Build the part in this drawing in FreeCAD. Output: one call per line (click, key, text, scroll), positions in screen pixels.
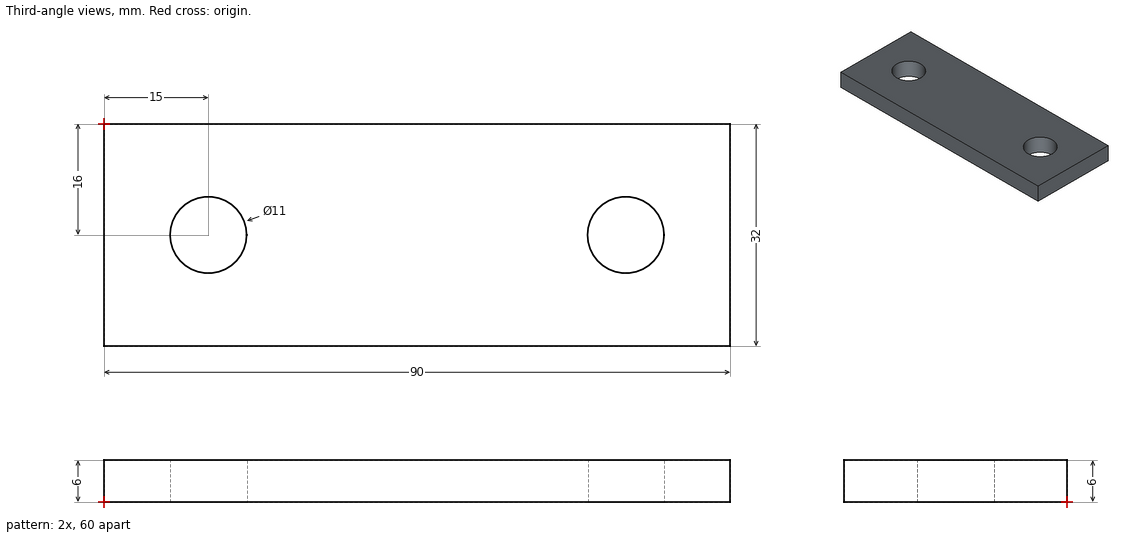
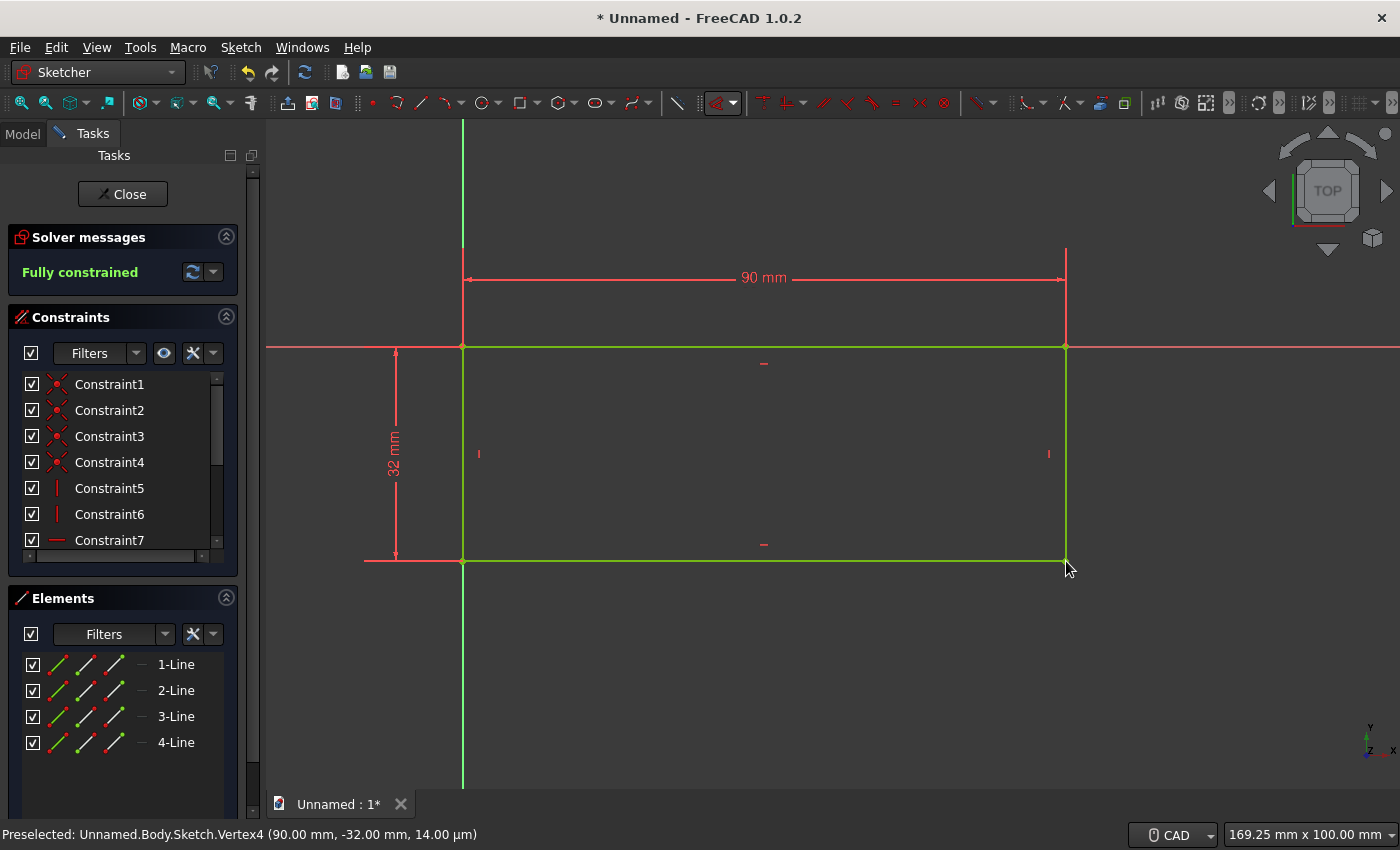
click(123, 194)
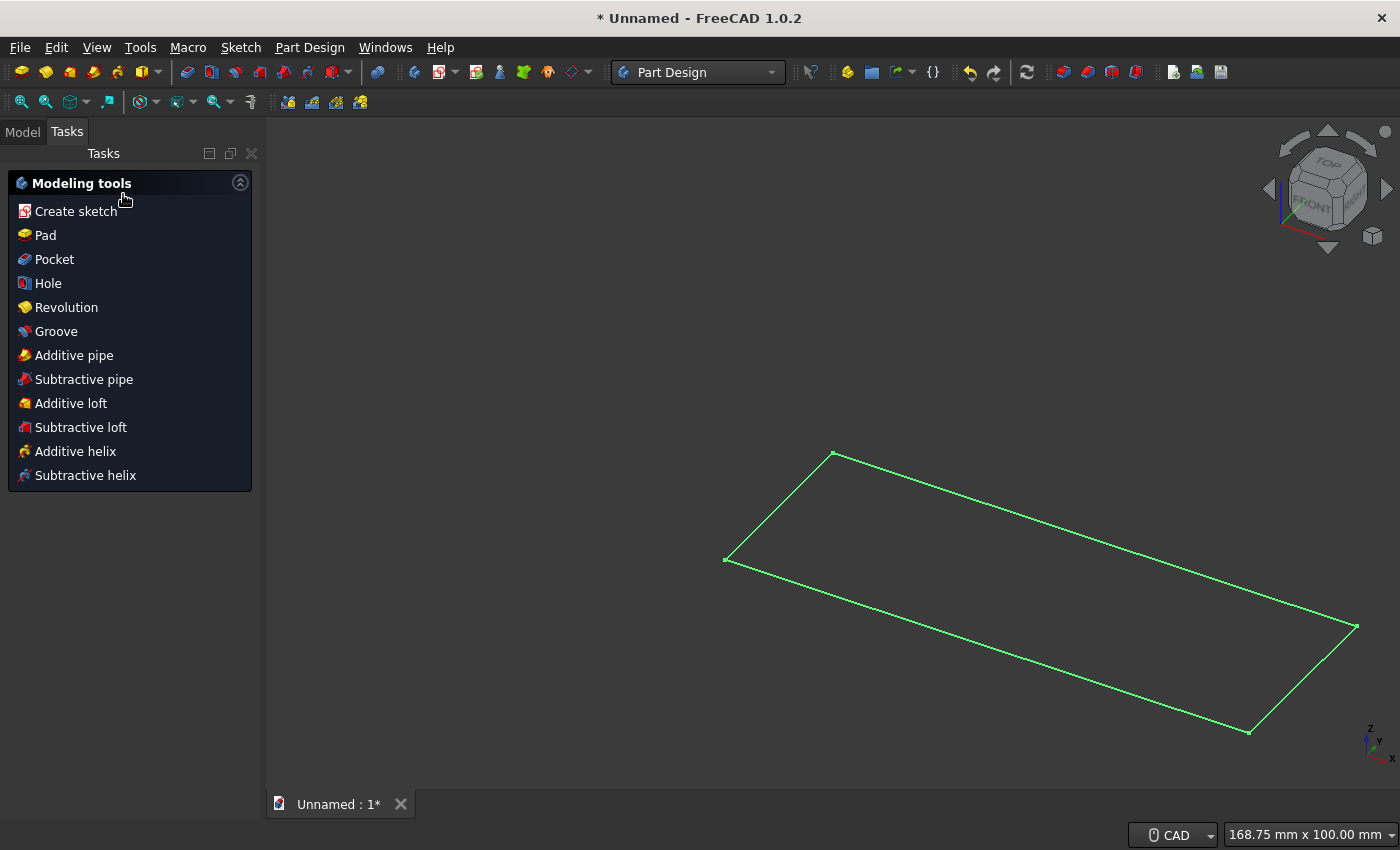
click(22, 72)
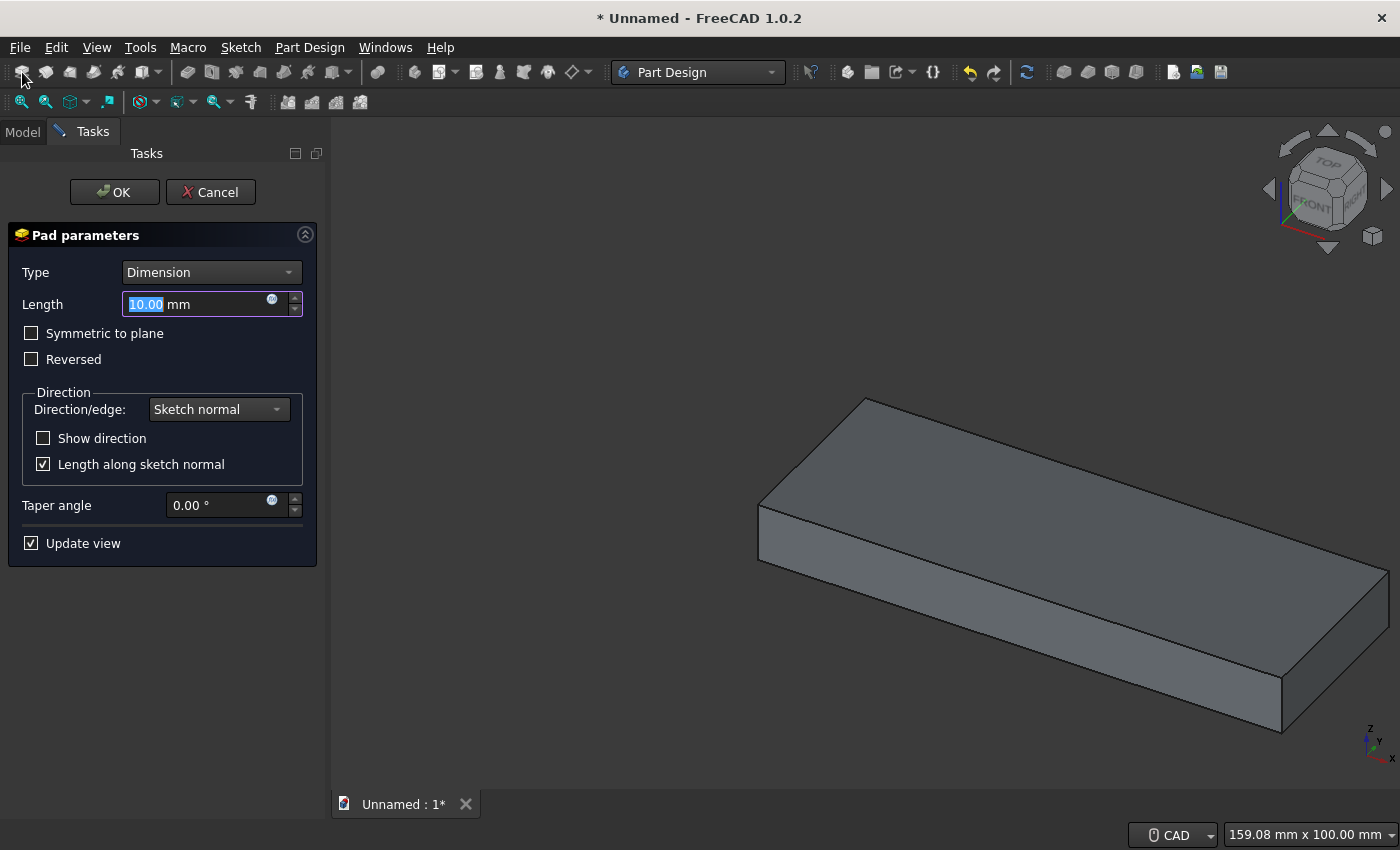
text(6)
key(Tab)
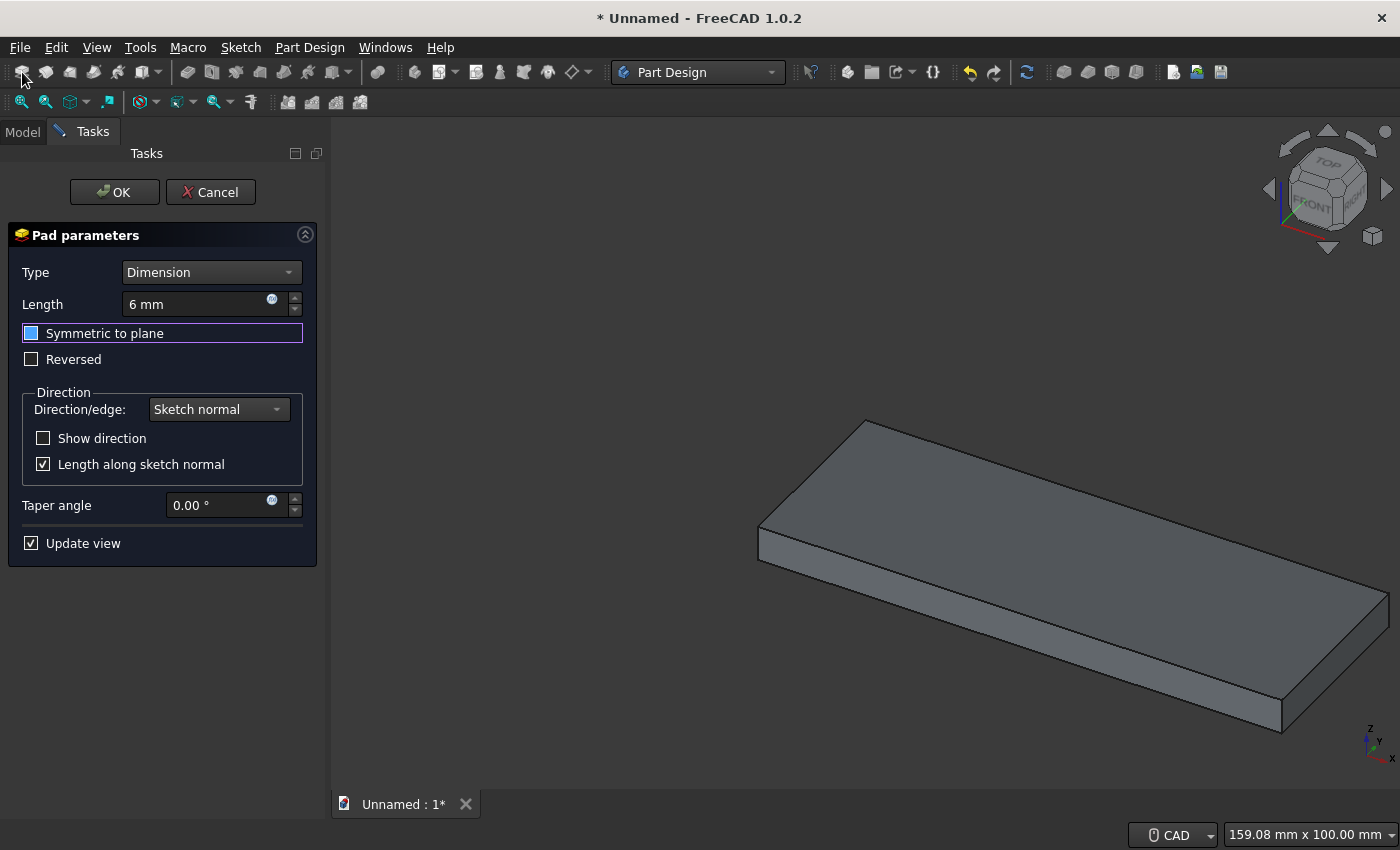
click(115, 192)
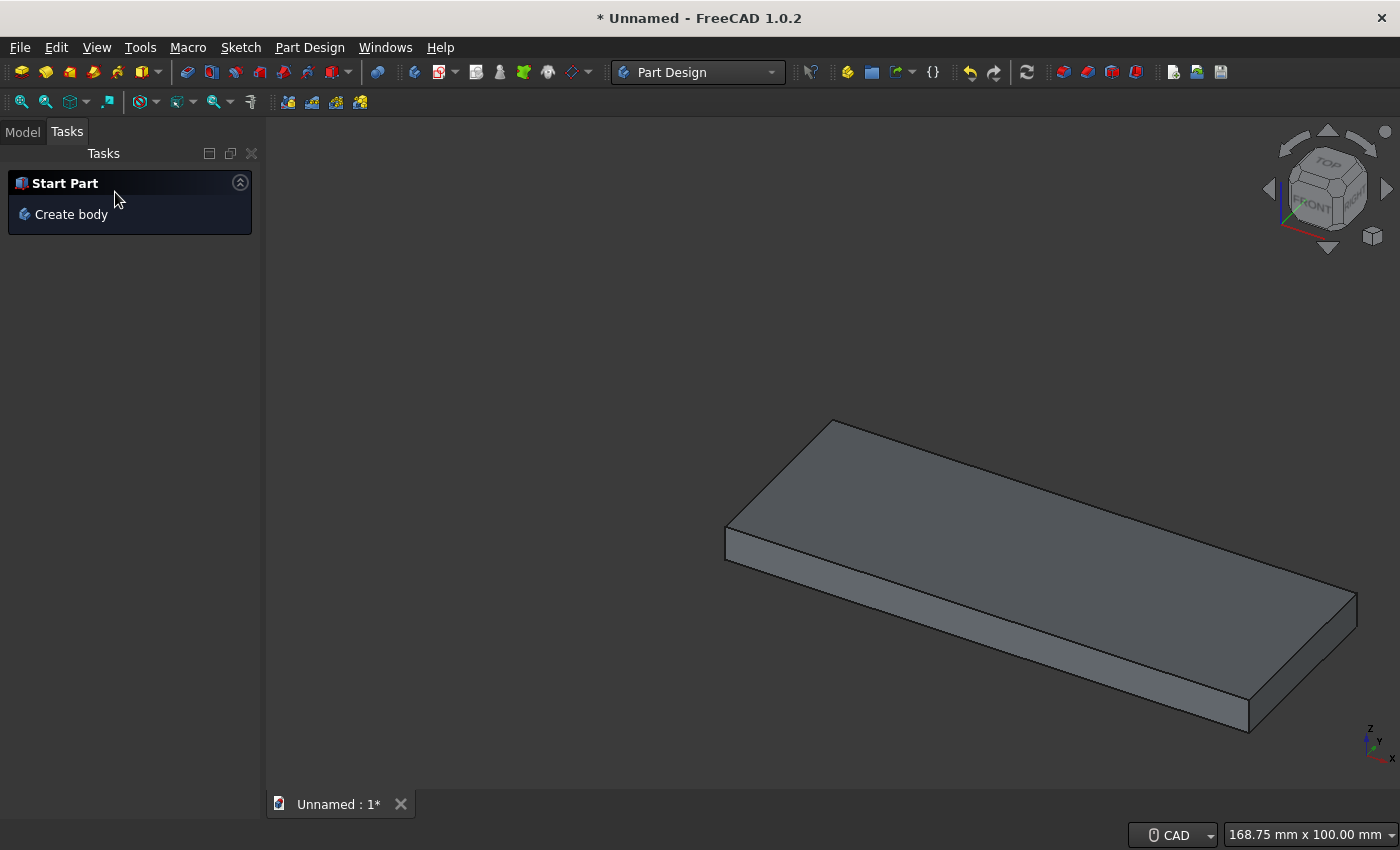
click(1191, 609)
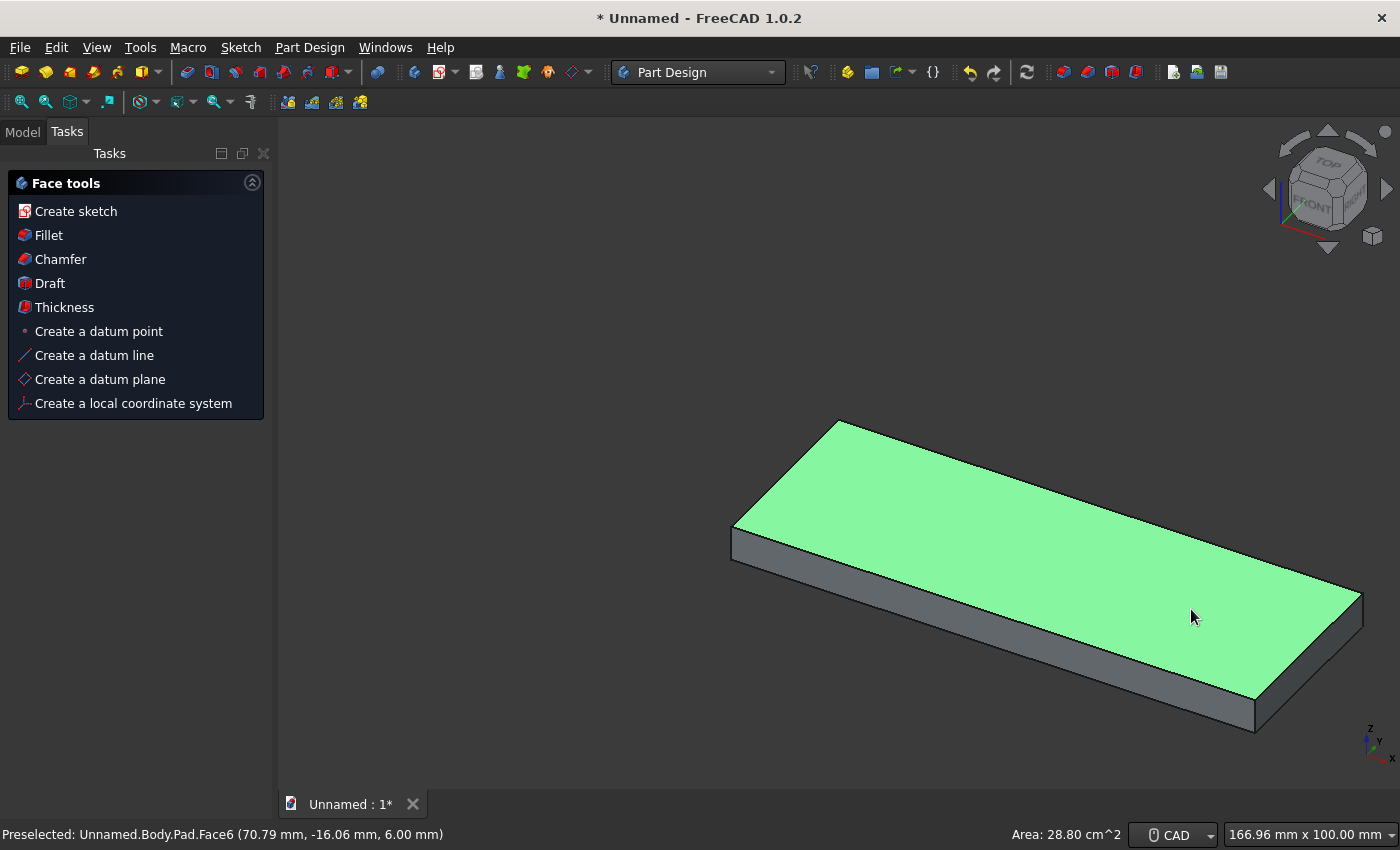
click(440, 72)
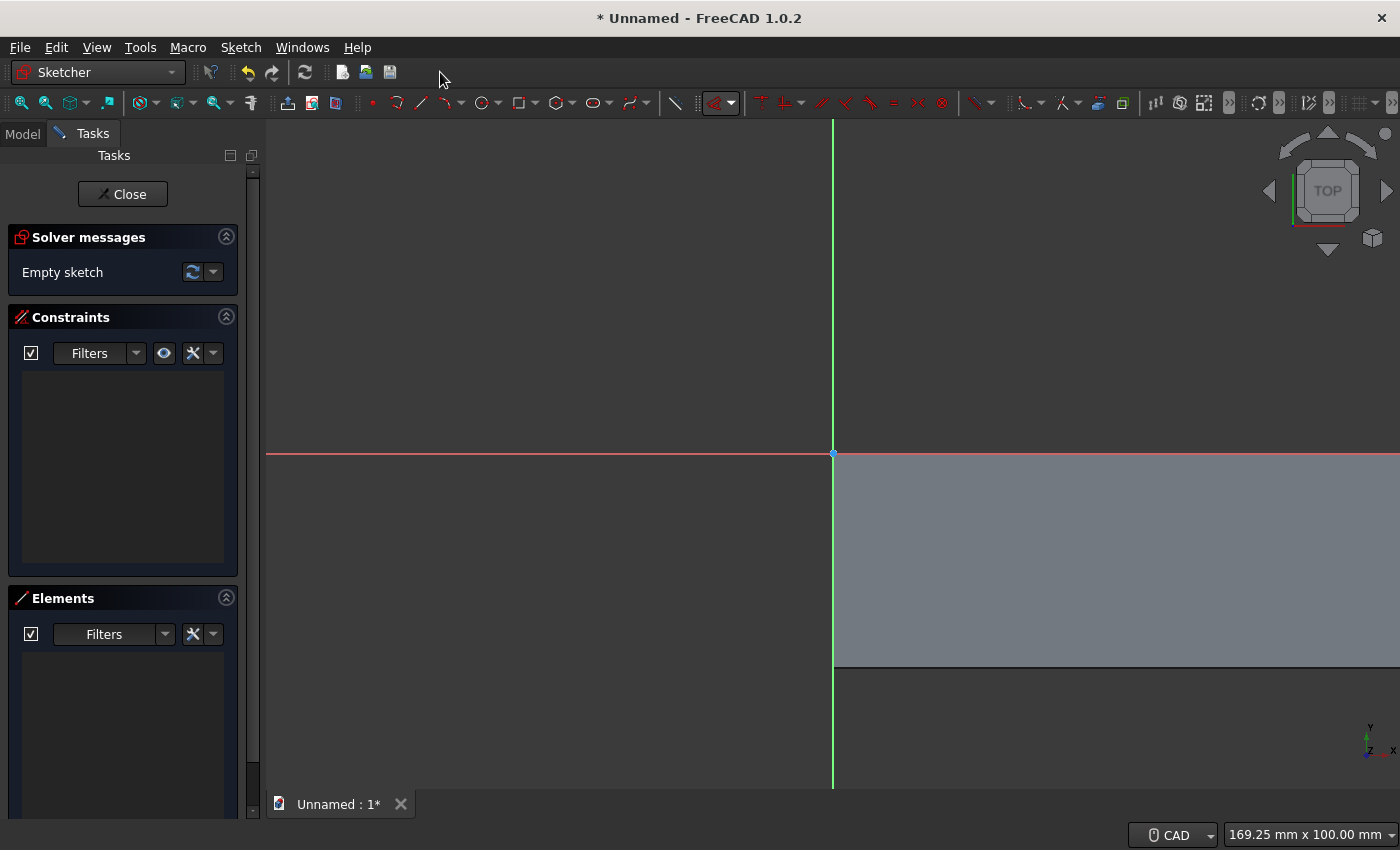
scroll(961, 557, up, 6)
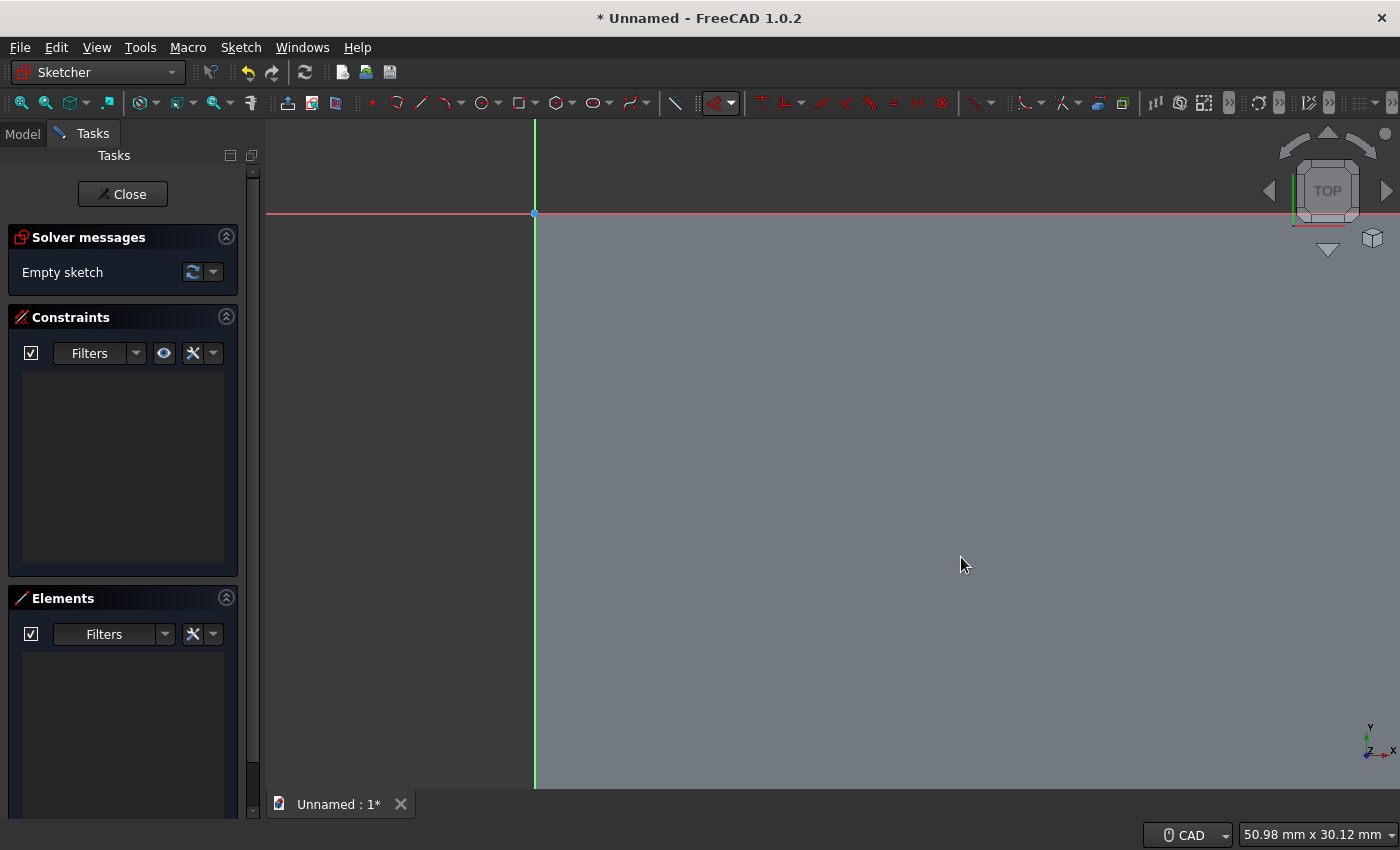
click(482, 104)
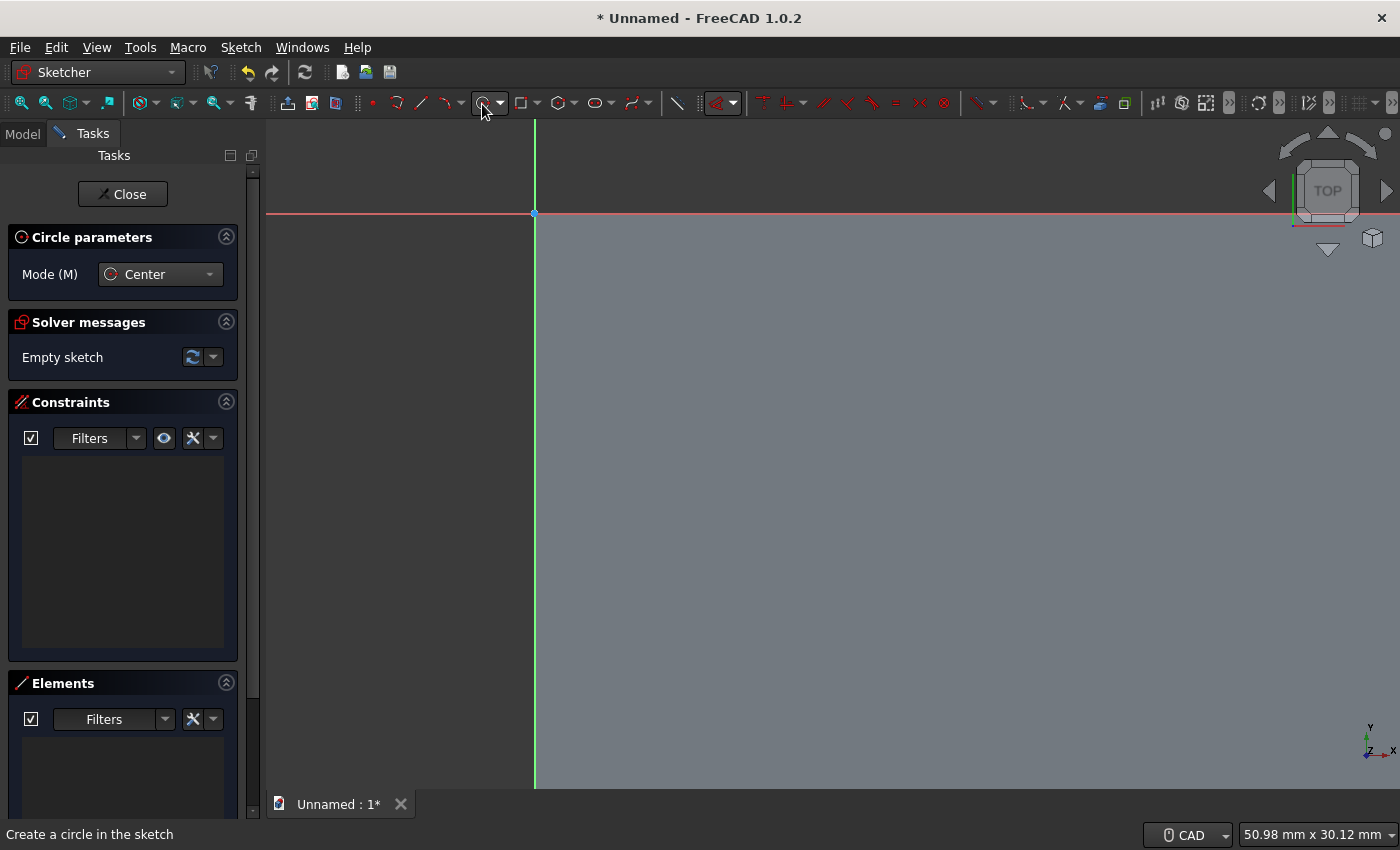
click(868, 569)
move(955, 483)